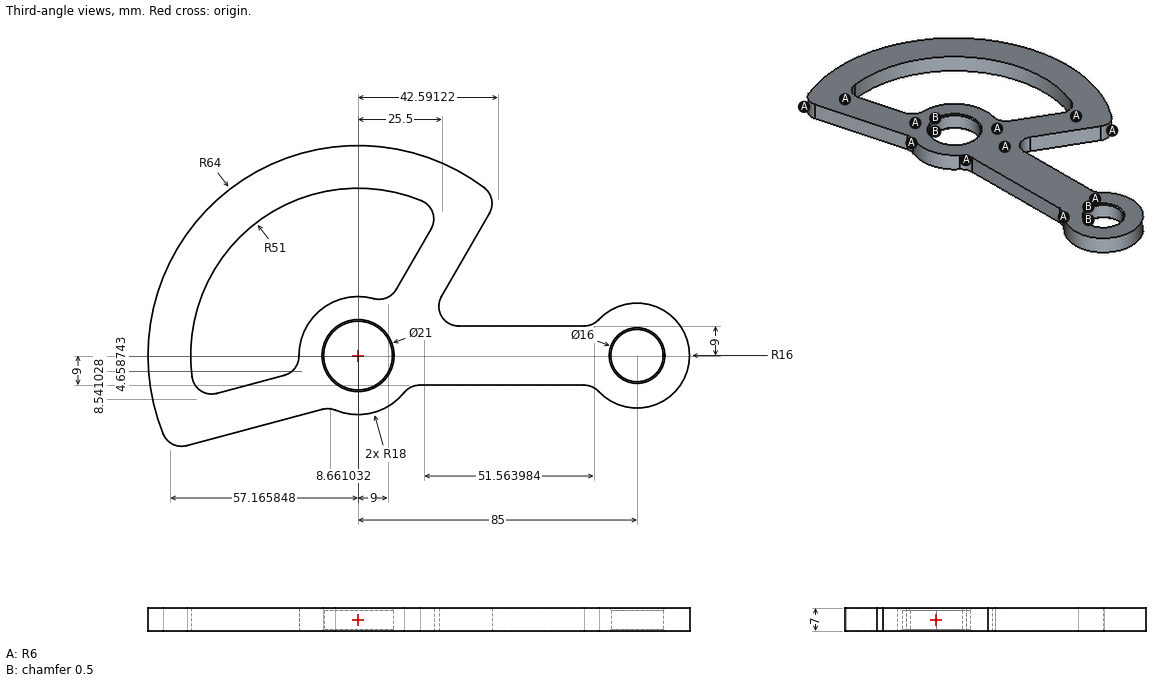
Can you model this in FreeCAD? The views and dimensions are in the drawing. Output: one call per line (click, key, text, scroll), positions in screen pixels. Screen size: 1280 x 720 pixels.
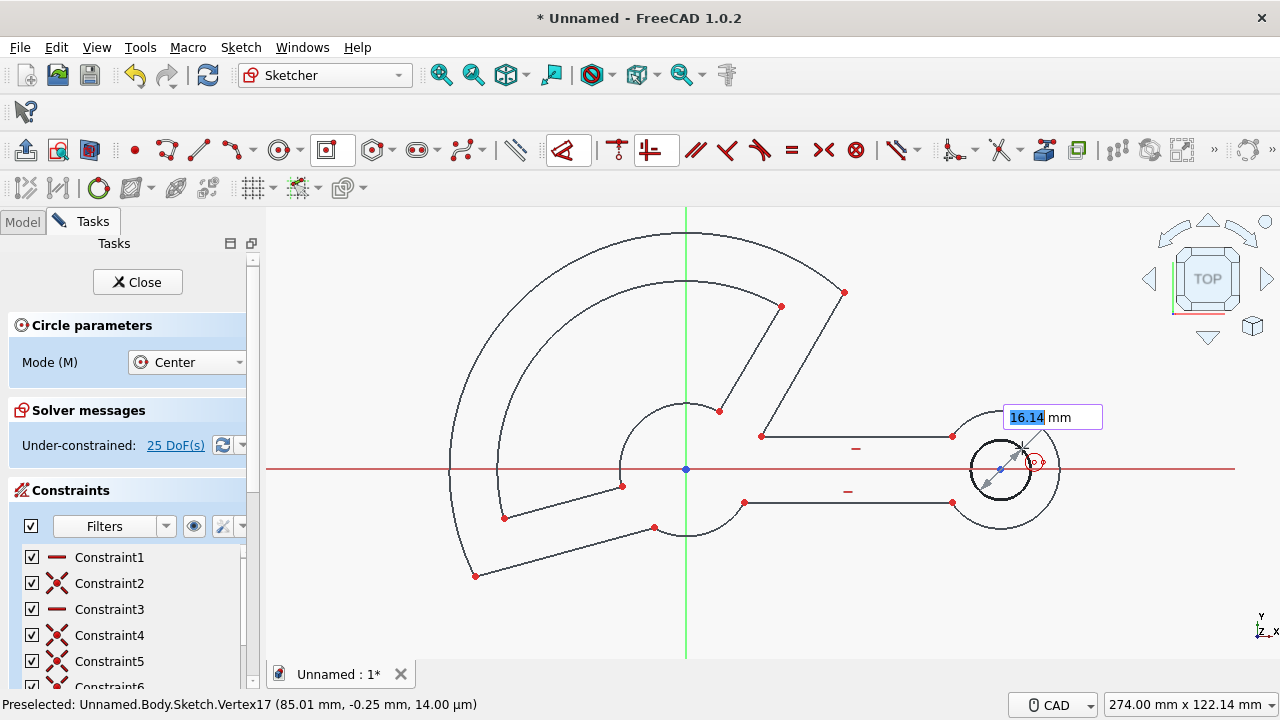
text(16)
key(Return)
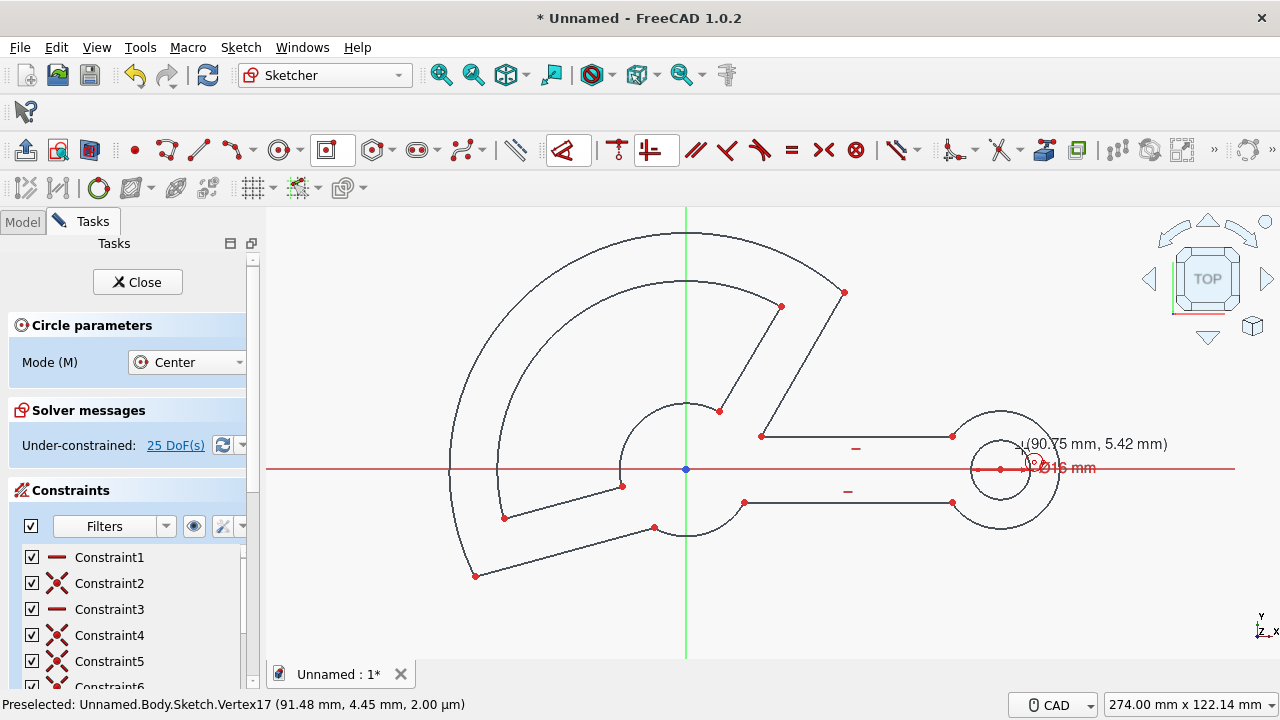
click(686, 469)
move(714, 442)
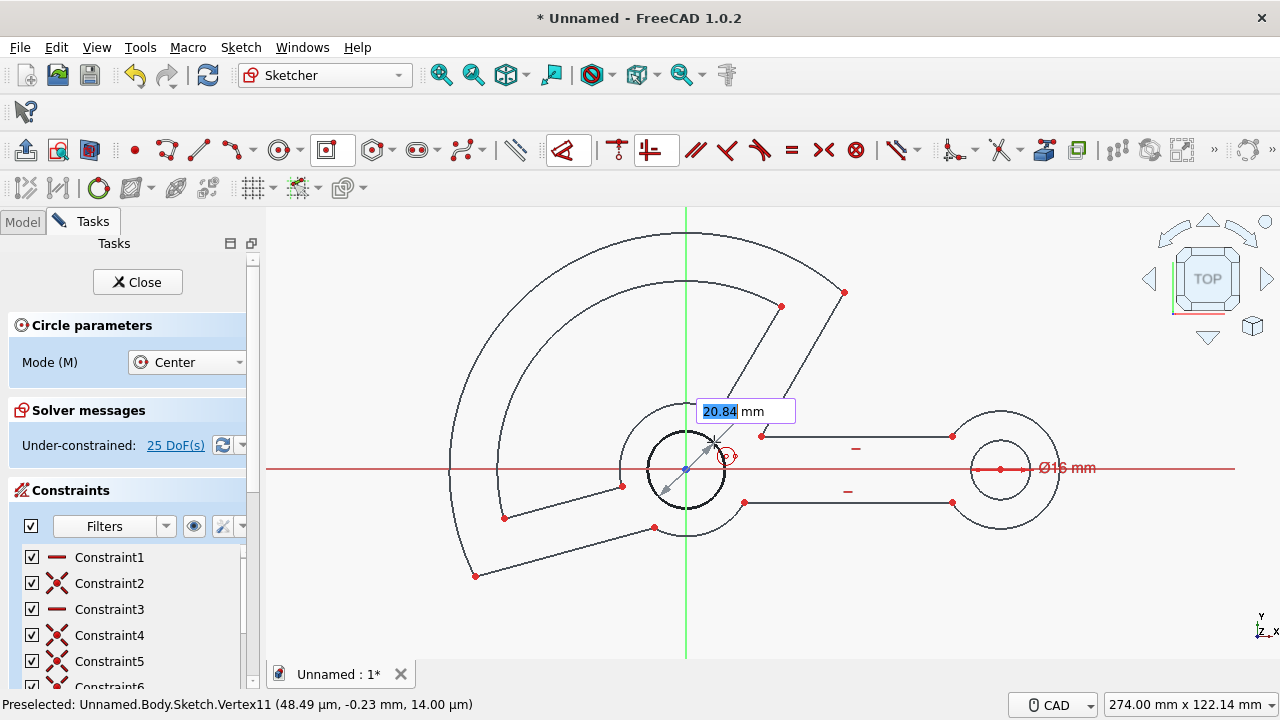
text(21)
key(Return)
key(Escape)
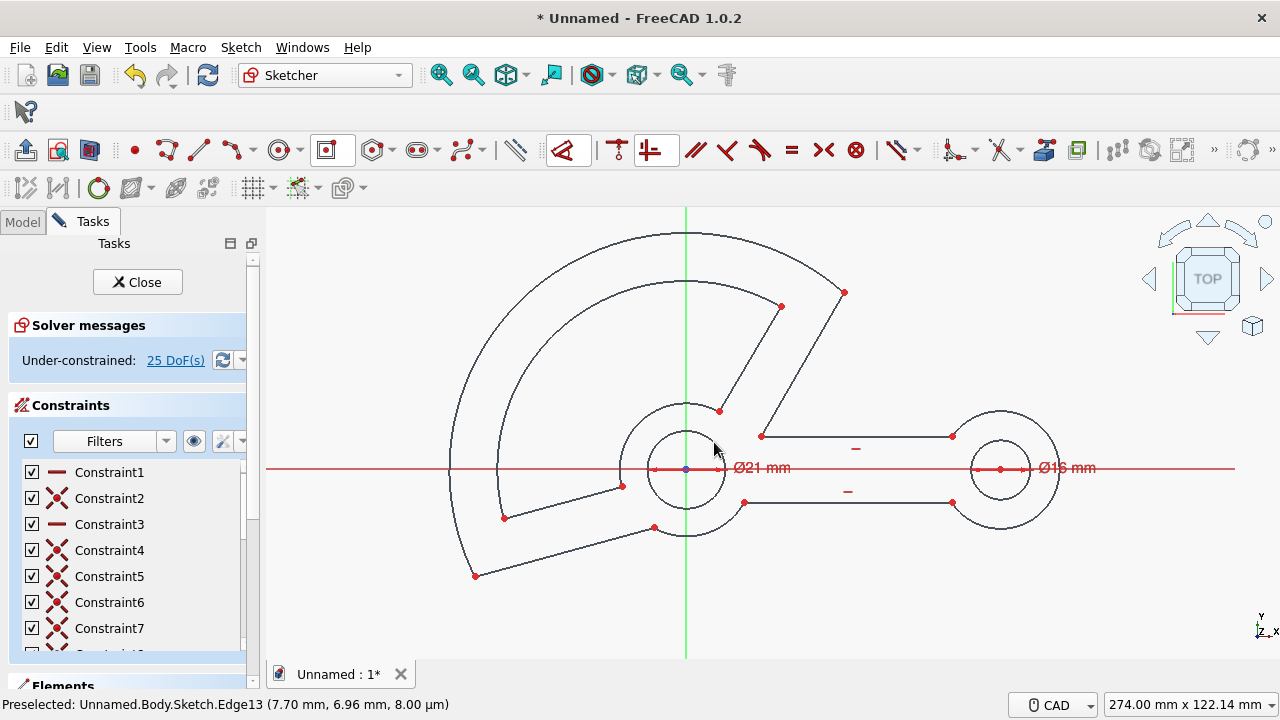
click(714, 442)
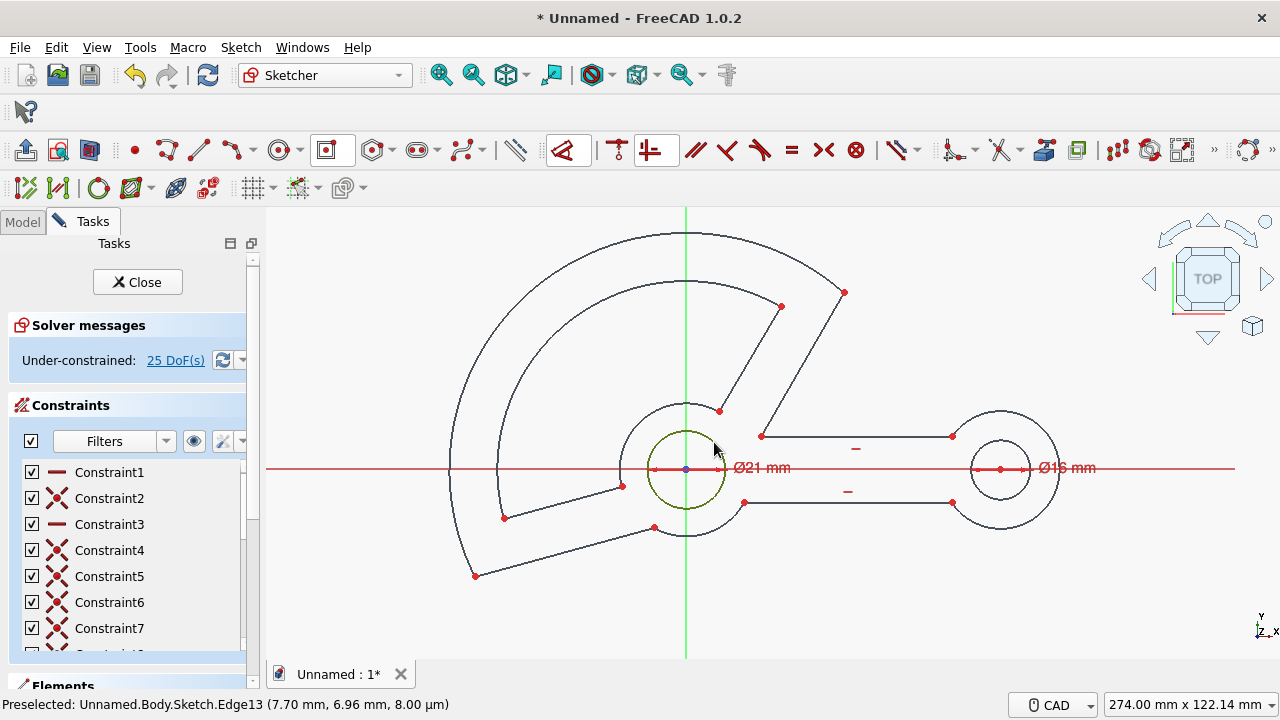
click(684, 536)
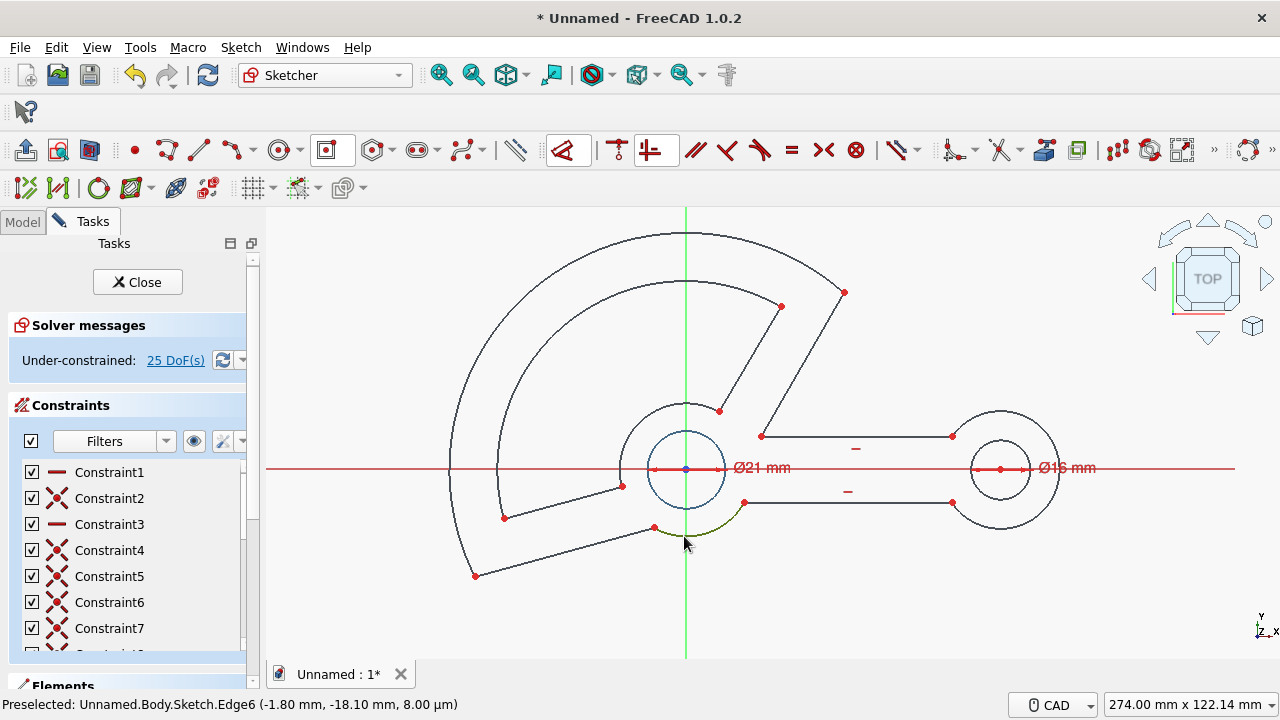
click(618, 150)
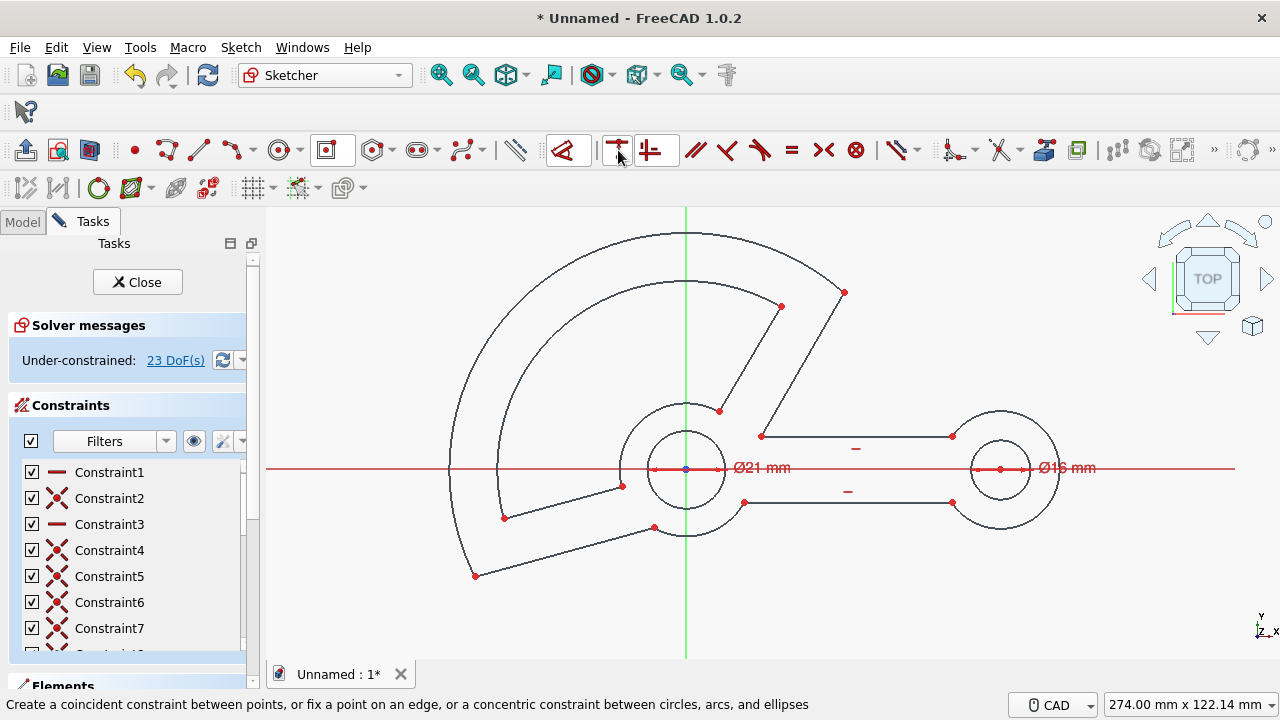
click(714, 442)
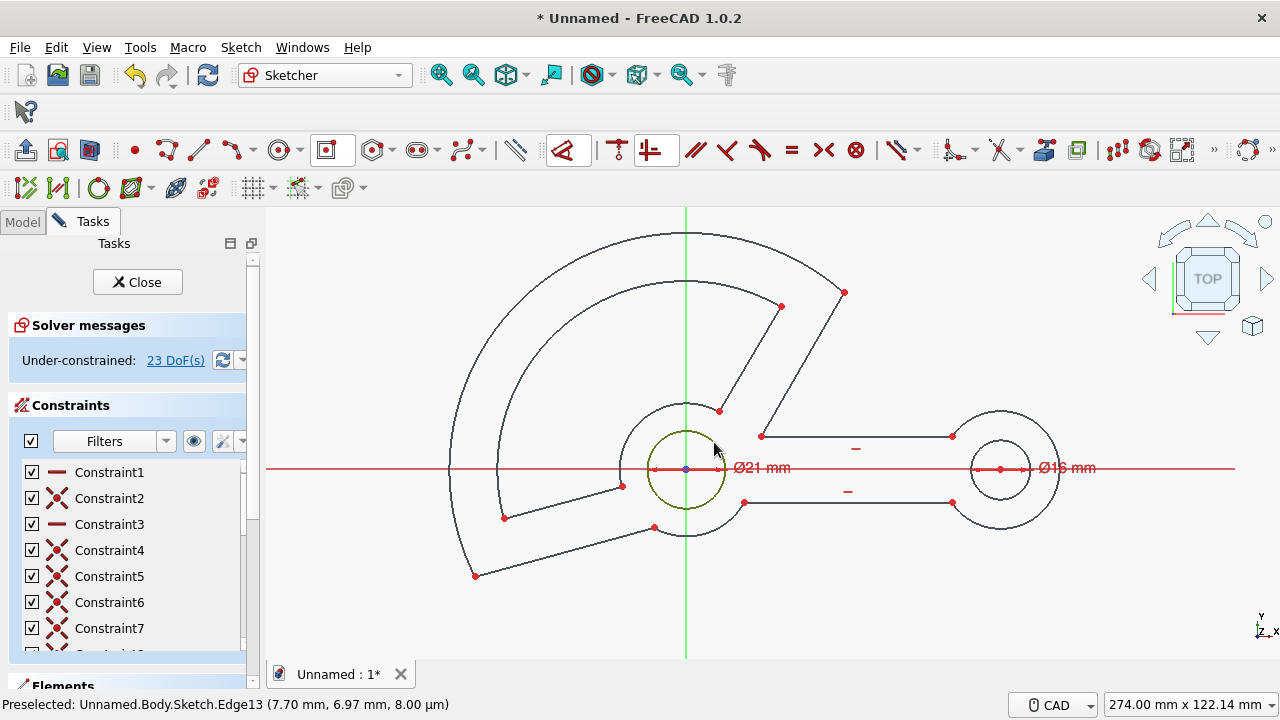
click(652, 284)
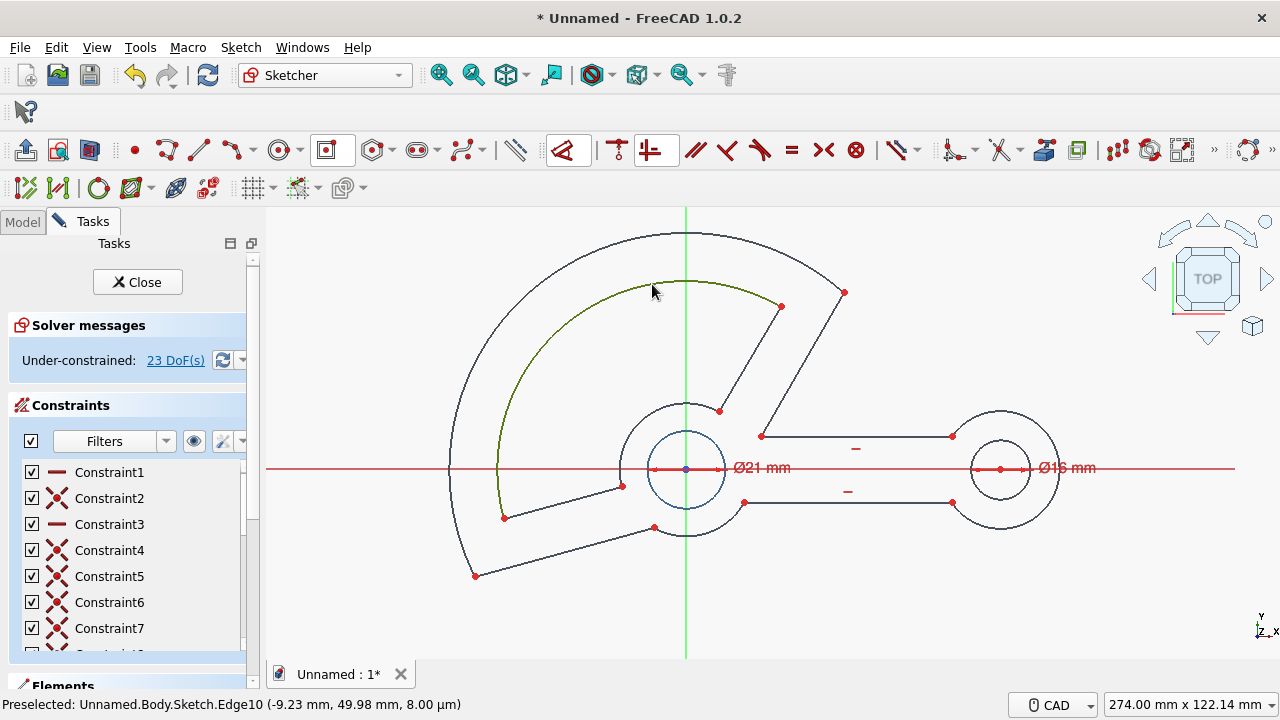
click(618, 150)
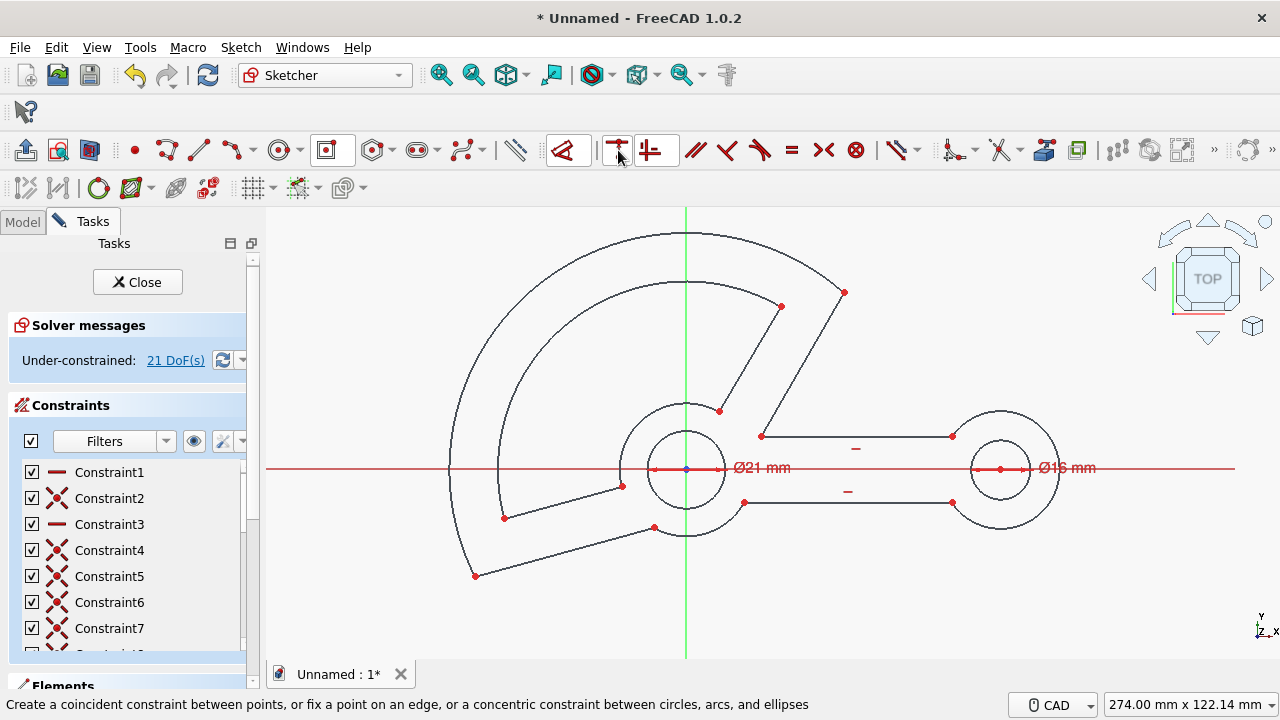
click(714, 442)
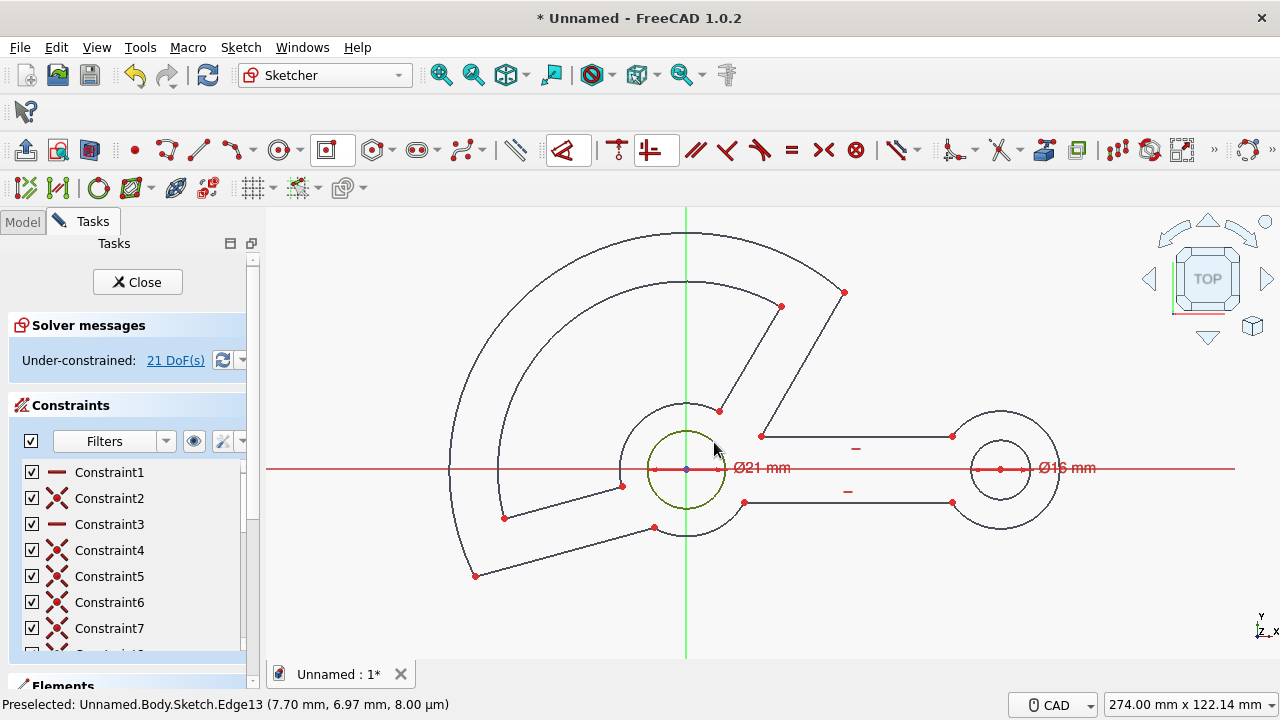
click(674, 405)